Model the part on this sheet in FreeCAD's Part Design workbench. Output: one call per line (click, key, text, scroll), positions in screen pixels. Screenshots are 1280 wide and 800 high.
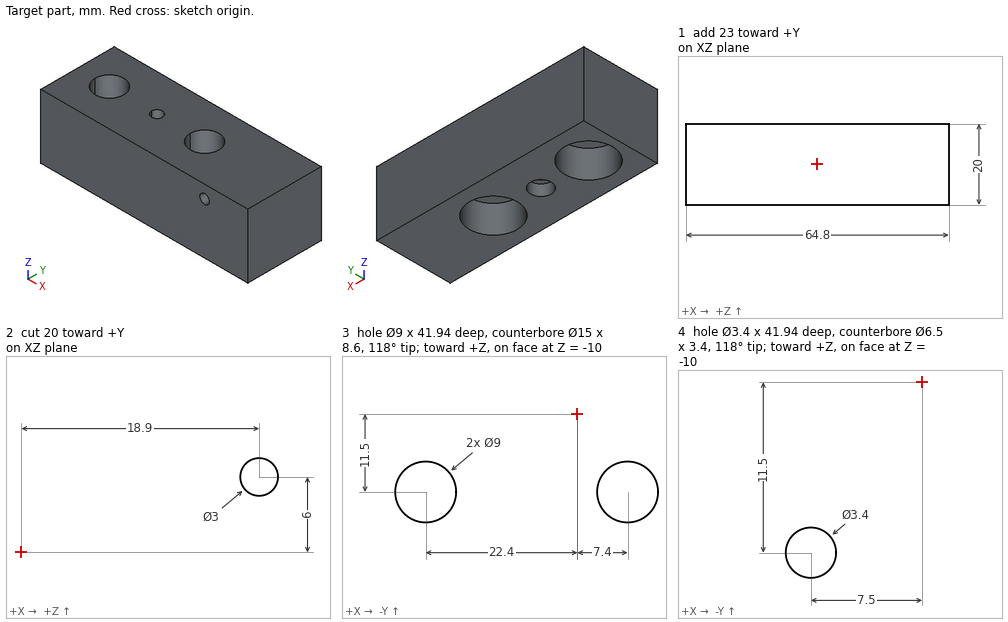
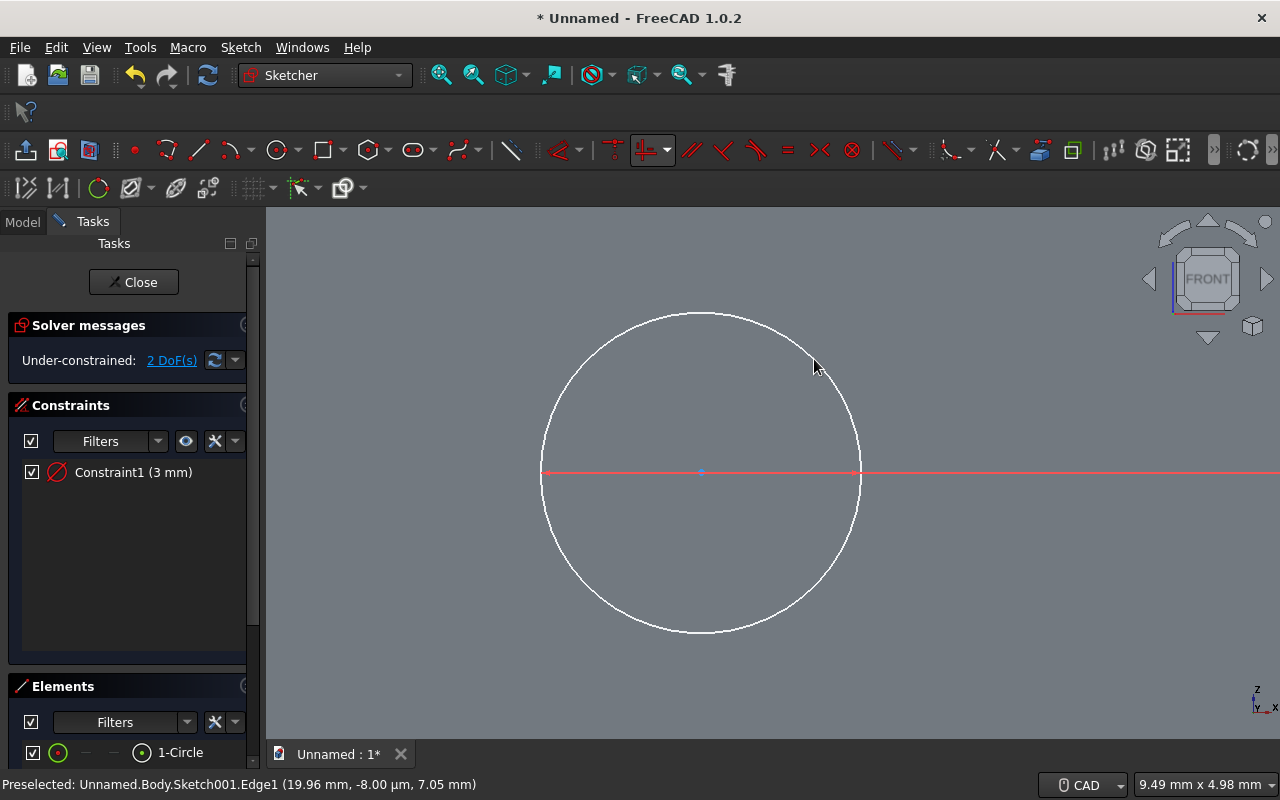
click(701, 473)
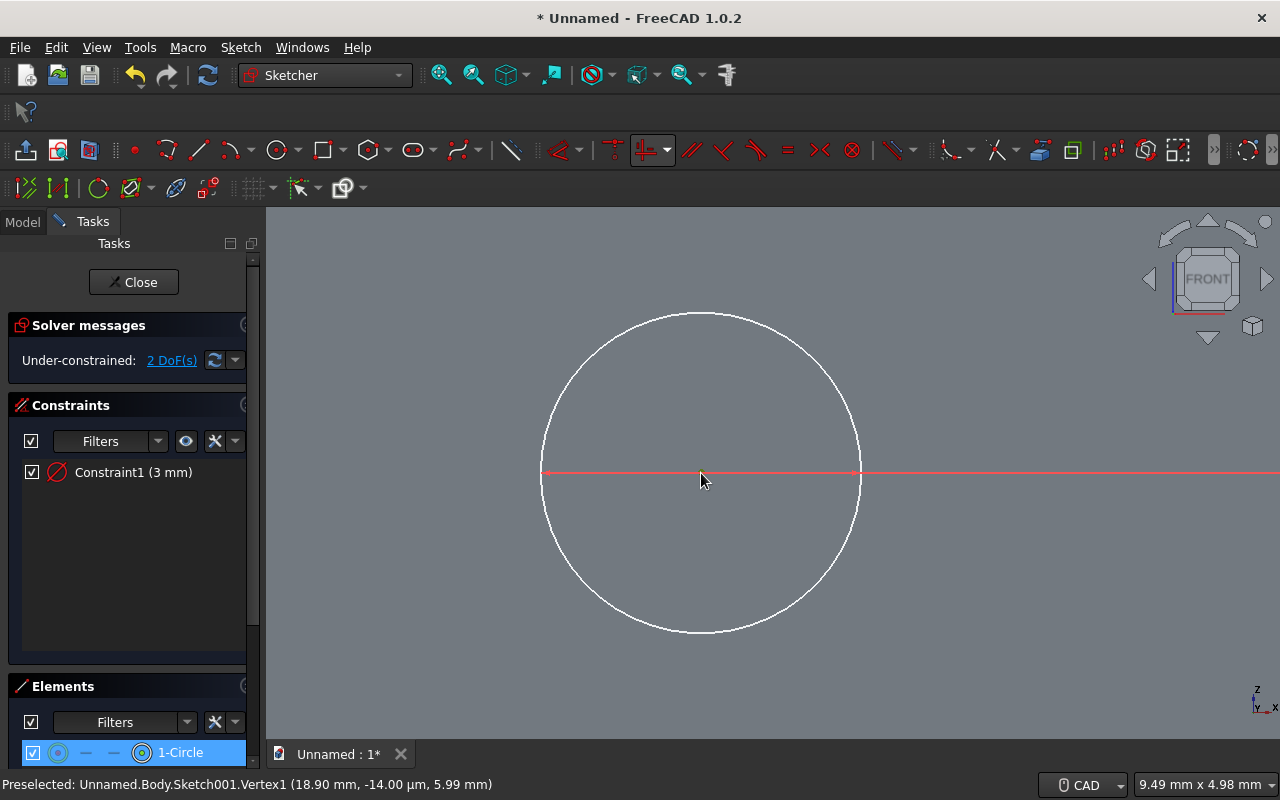
click(582, 150)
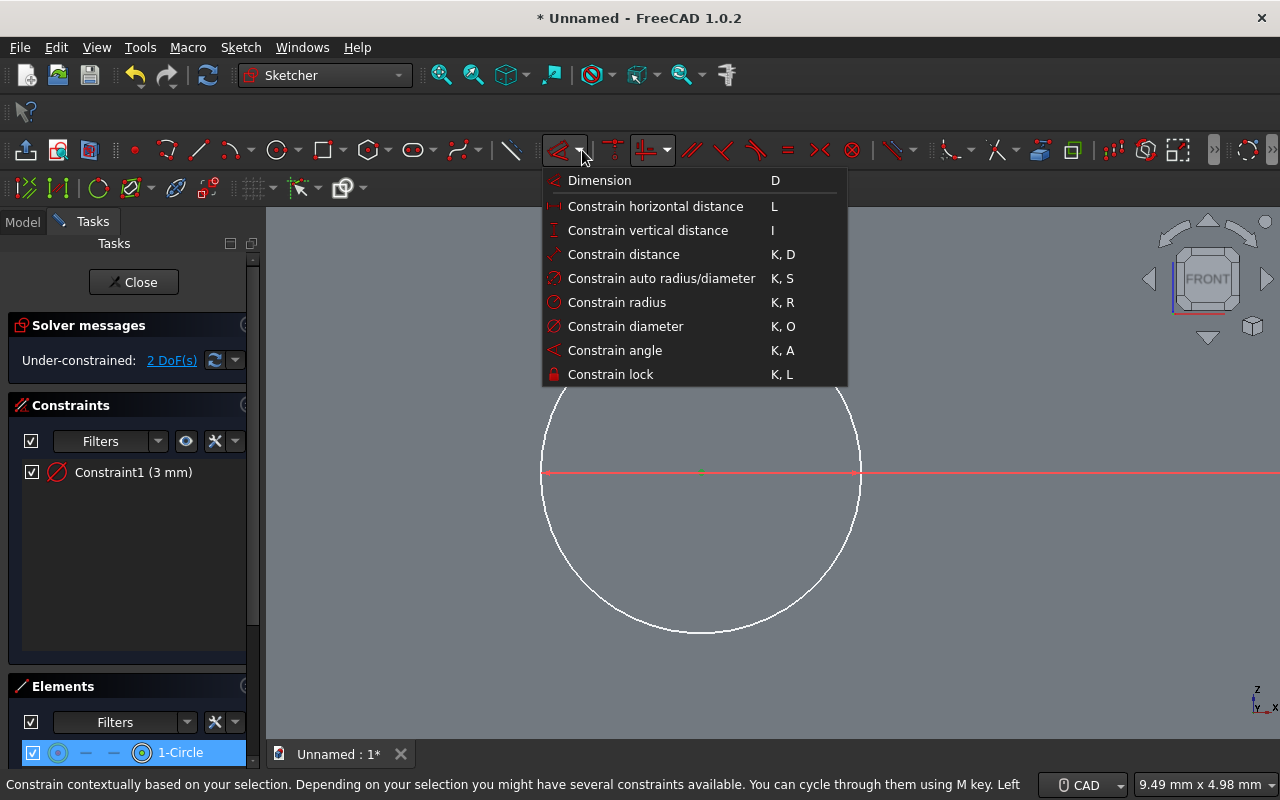
click(695, 230)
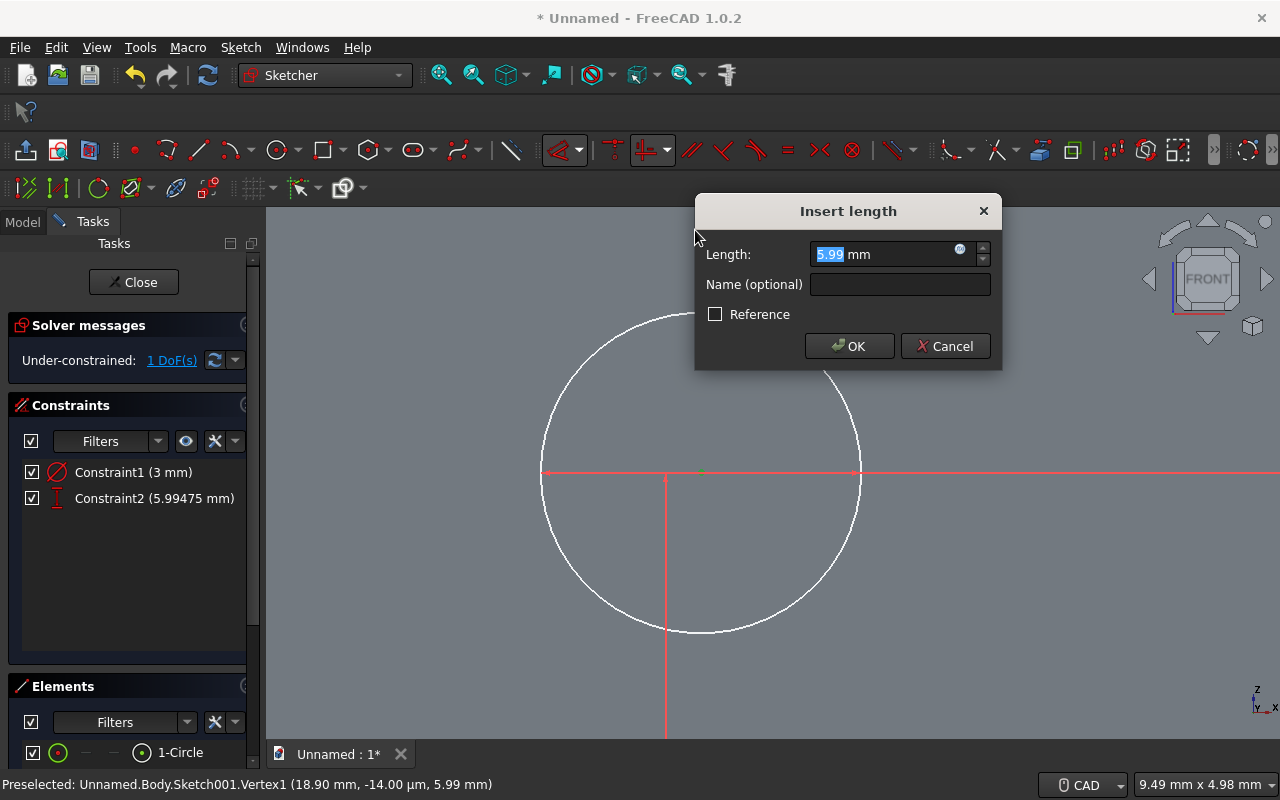
text(6)
key(Return)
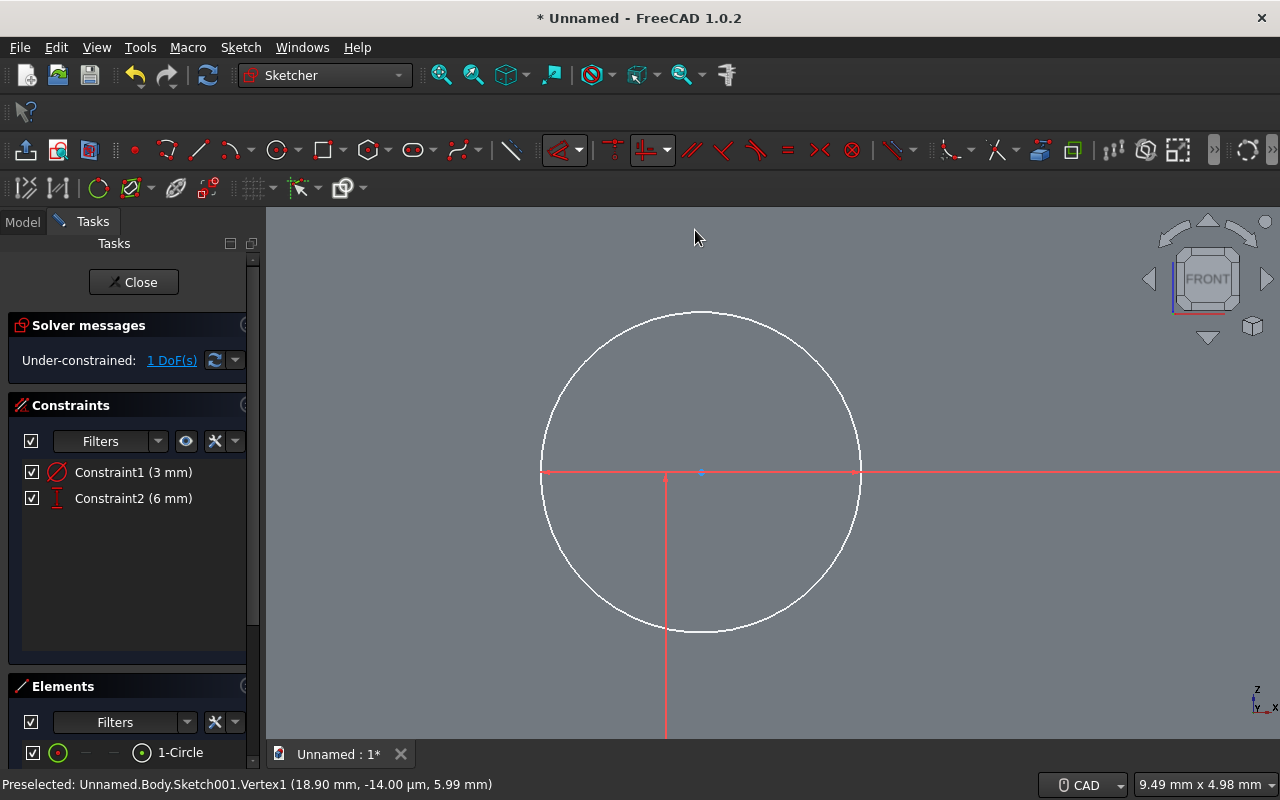
click(701, 472)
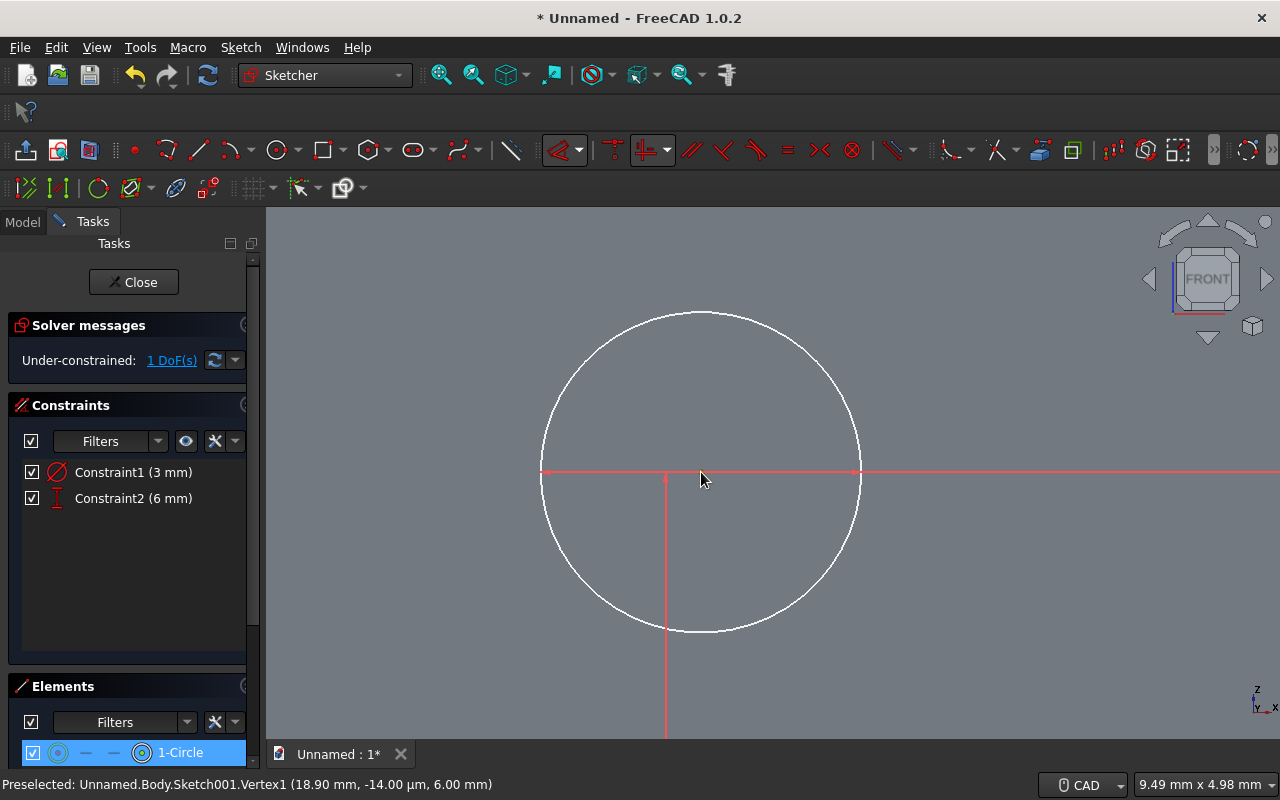
click(582, 150)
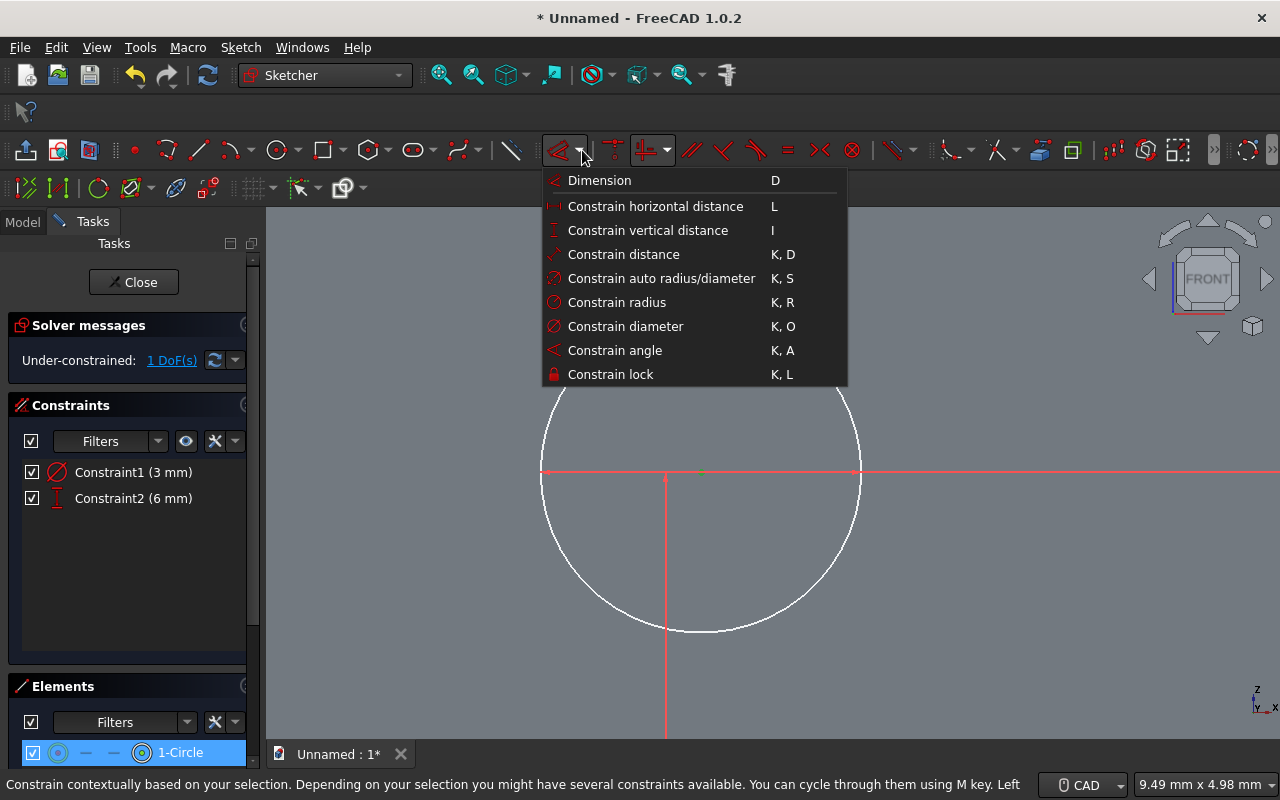
click(695, 206)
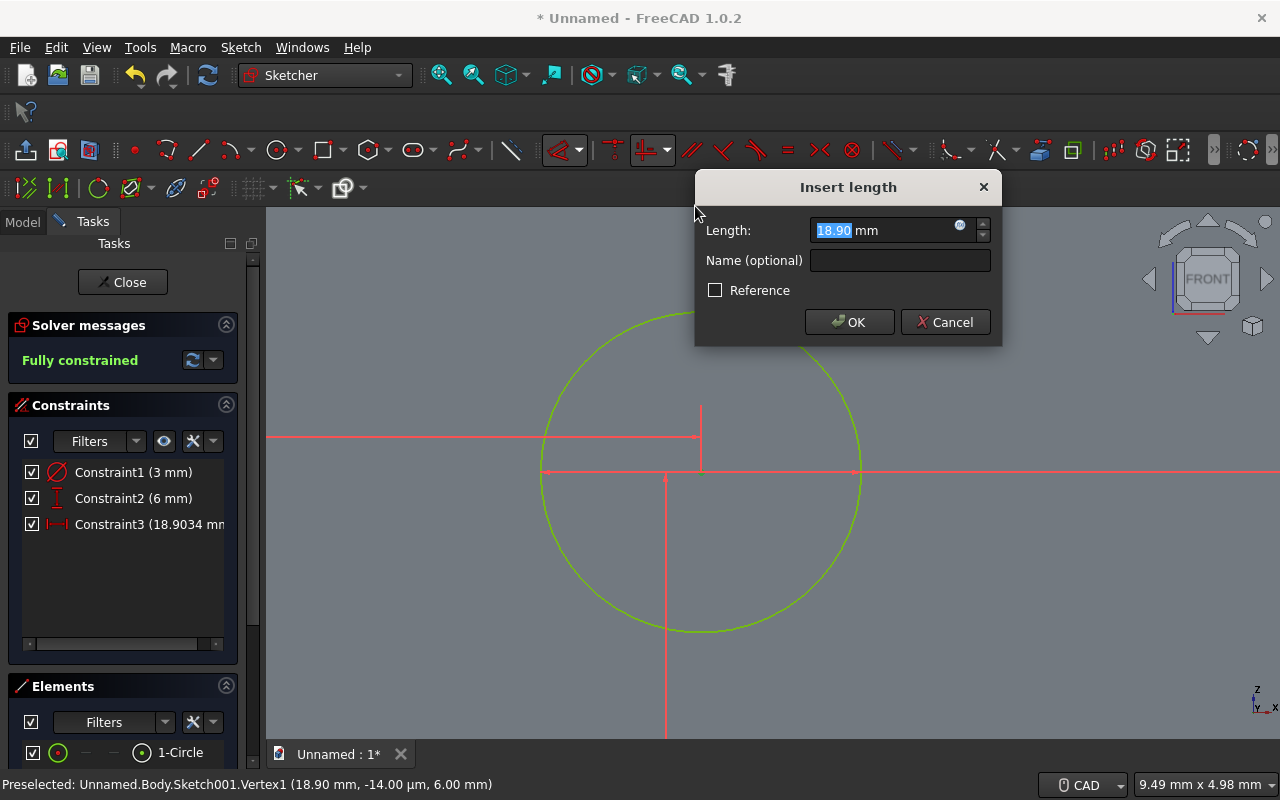
text(18.9)
key(Return)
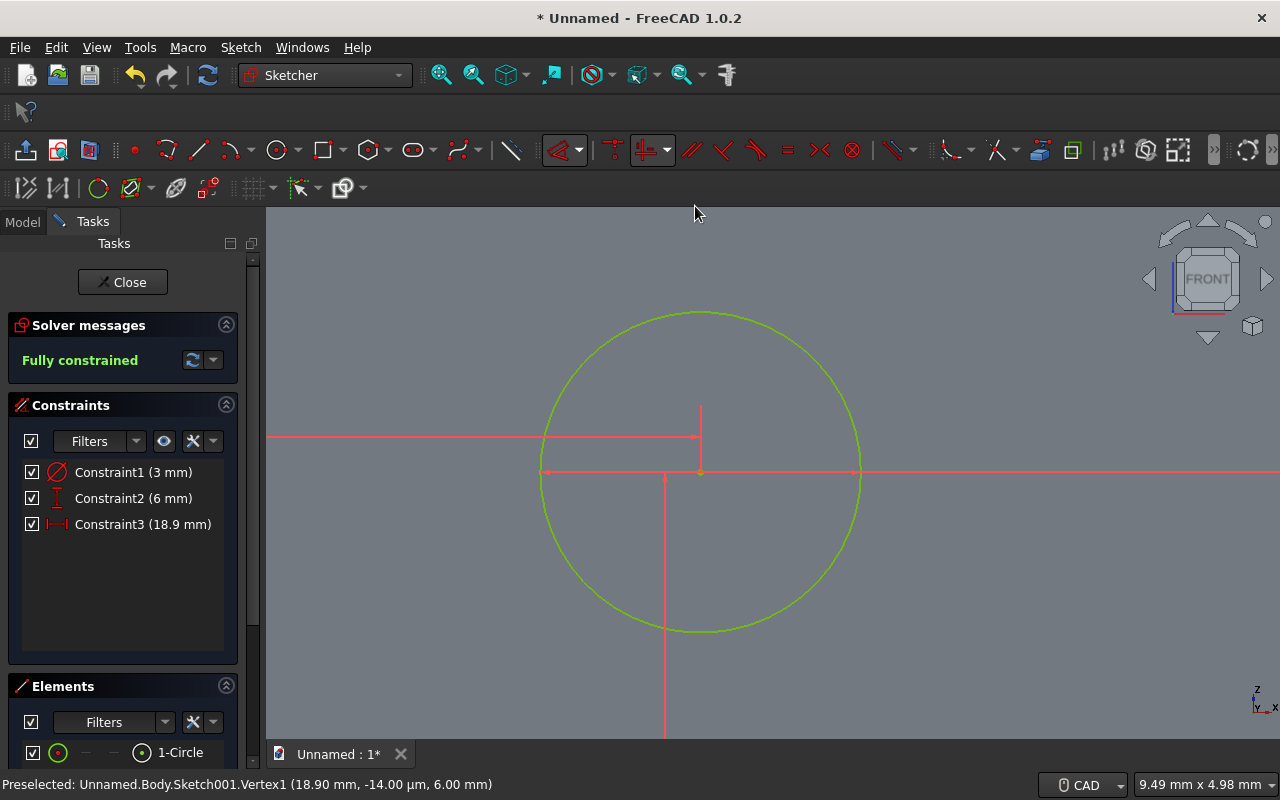
click(123, 282)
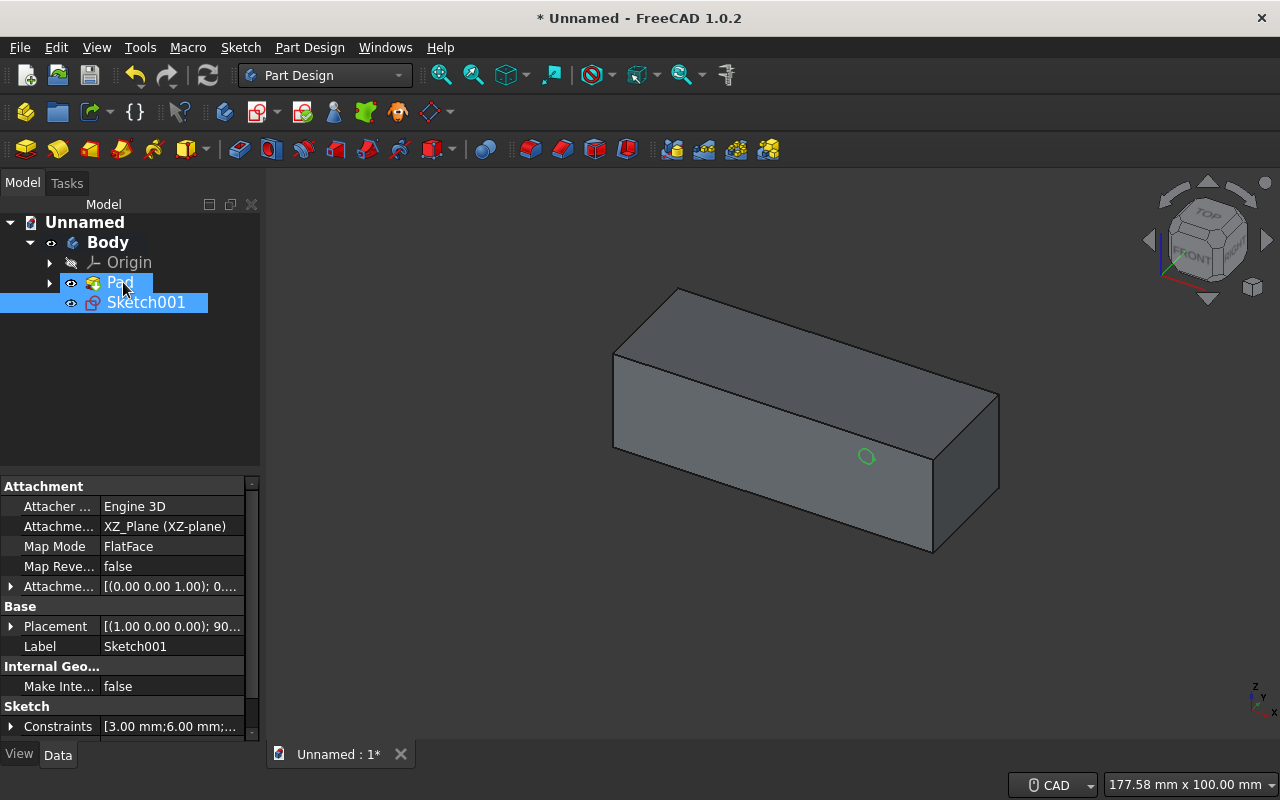
click(240, 150)